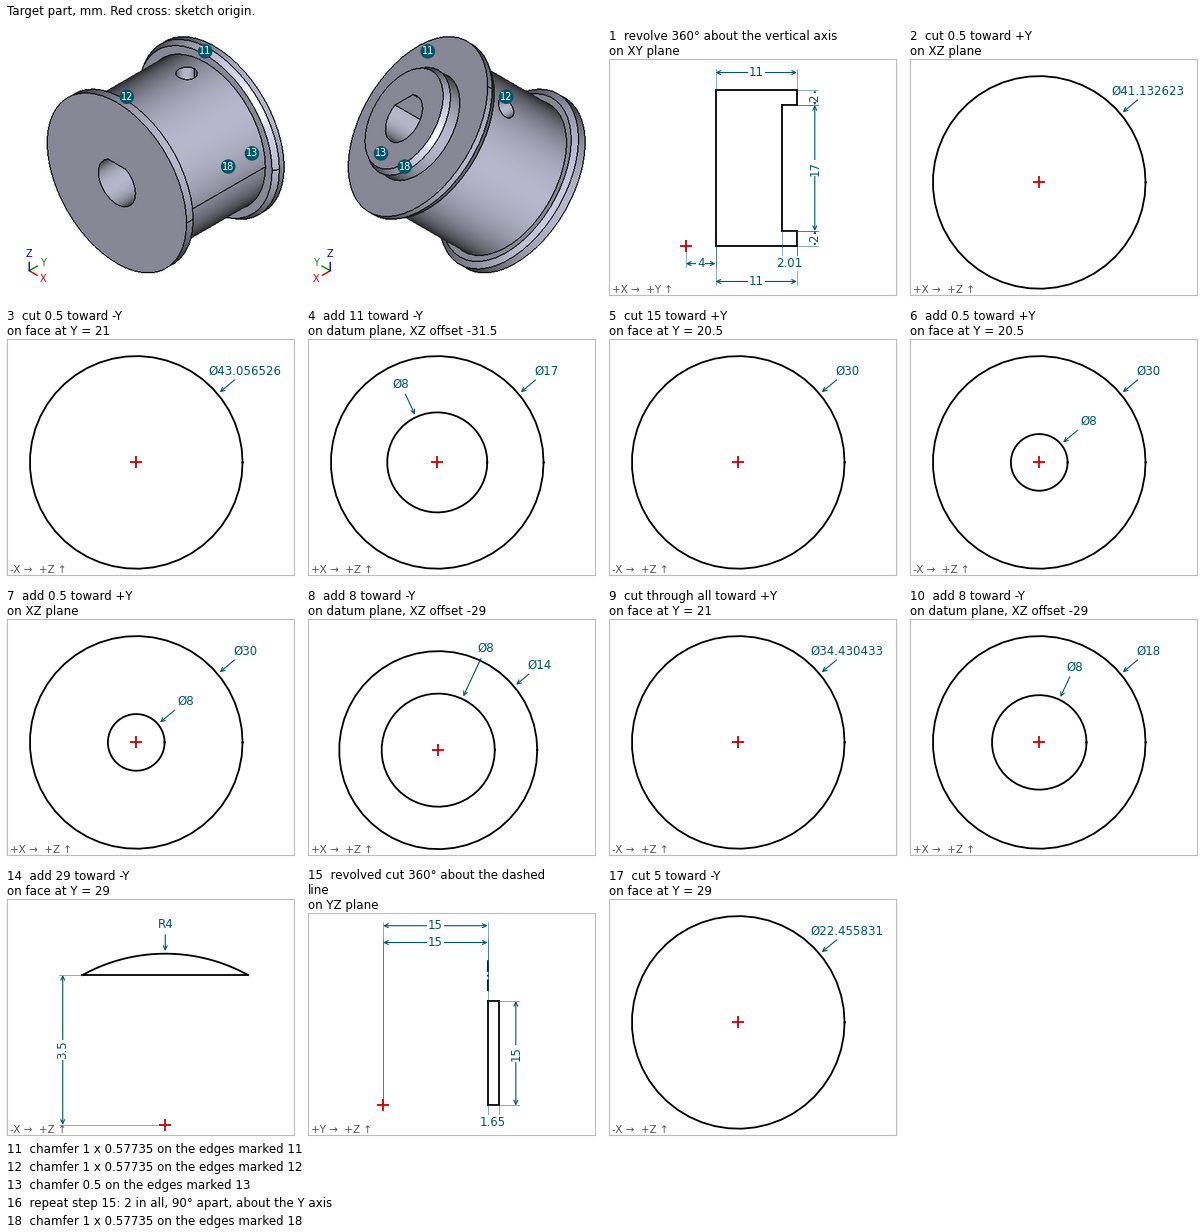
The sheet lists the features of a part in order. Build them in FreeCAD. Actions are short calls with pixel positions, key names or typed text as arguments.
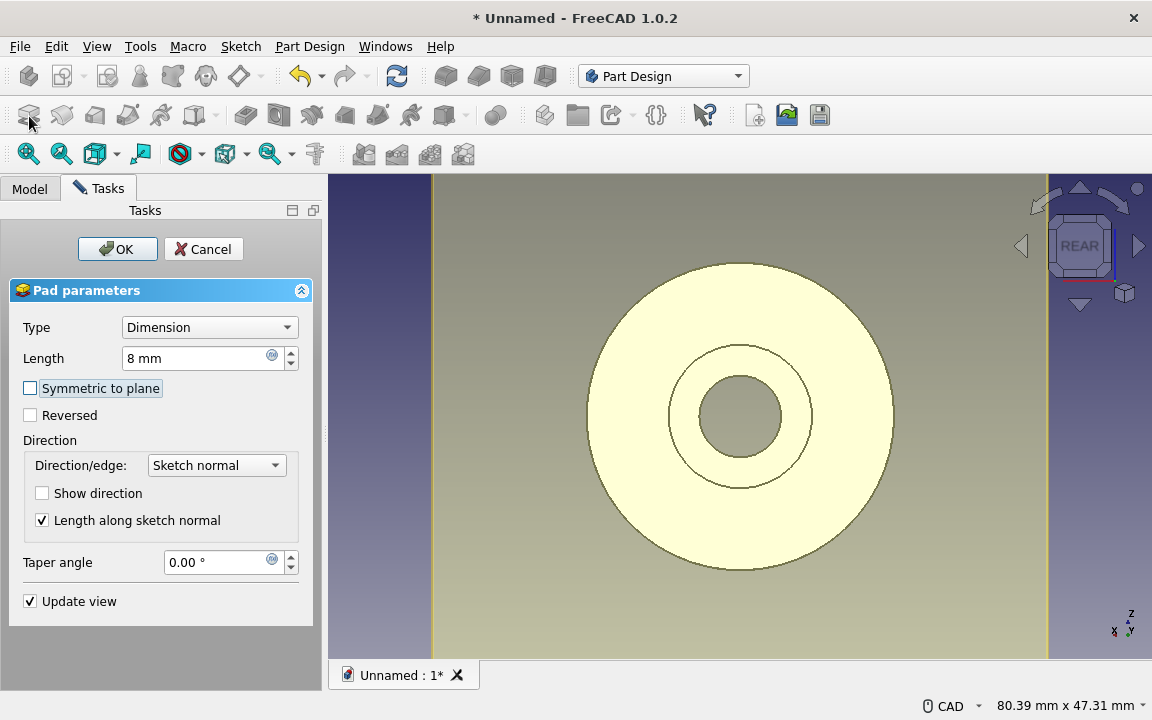
click(118, 249)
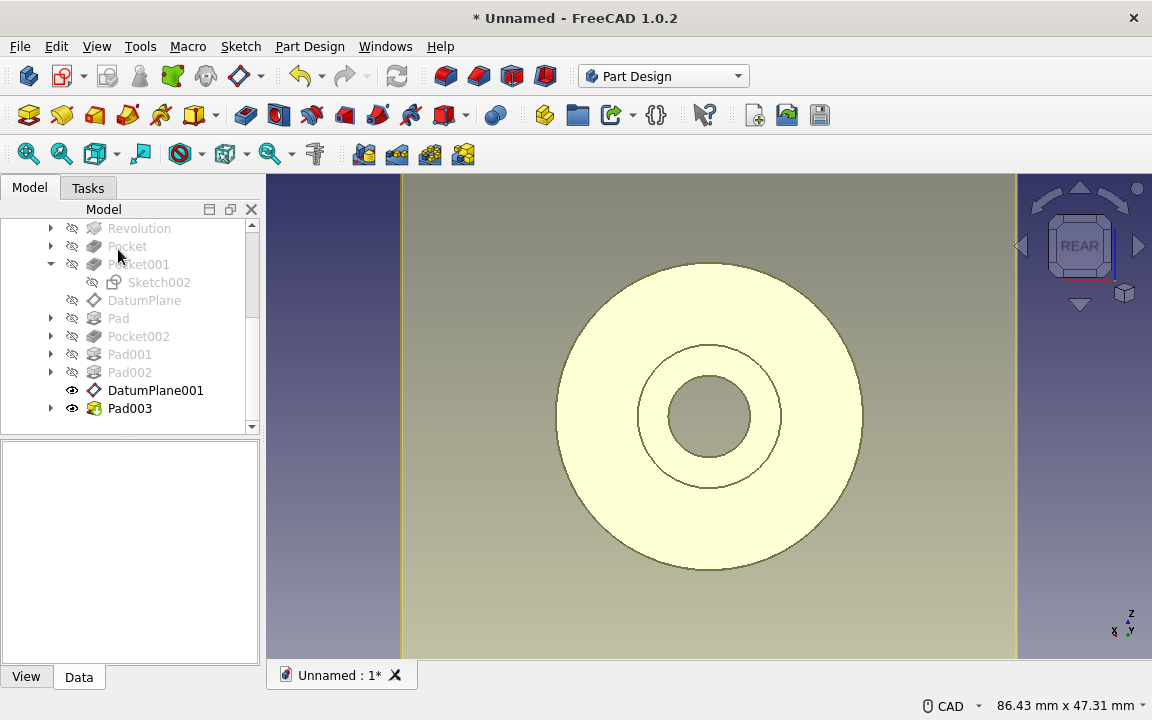
click(117, 390)
key(space)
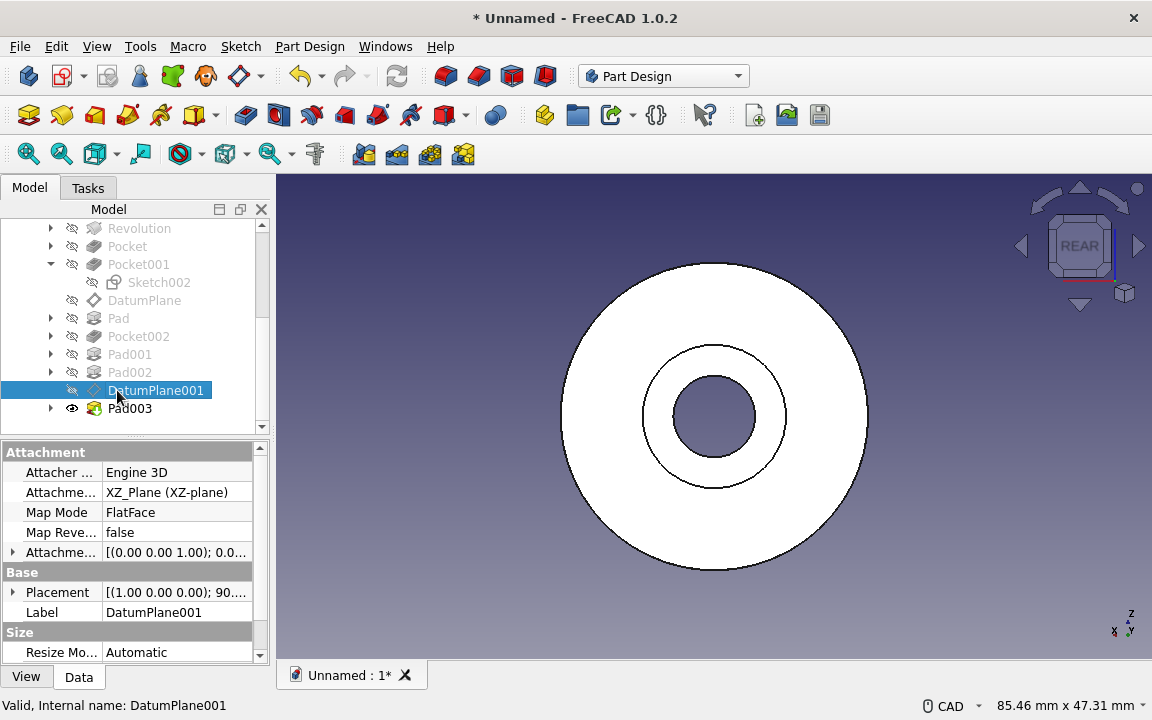
click(802, 503)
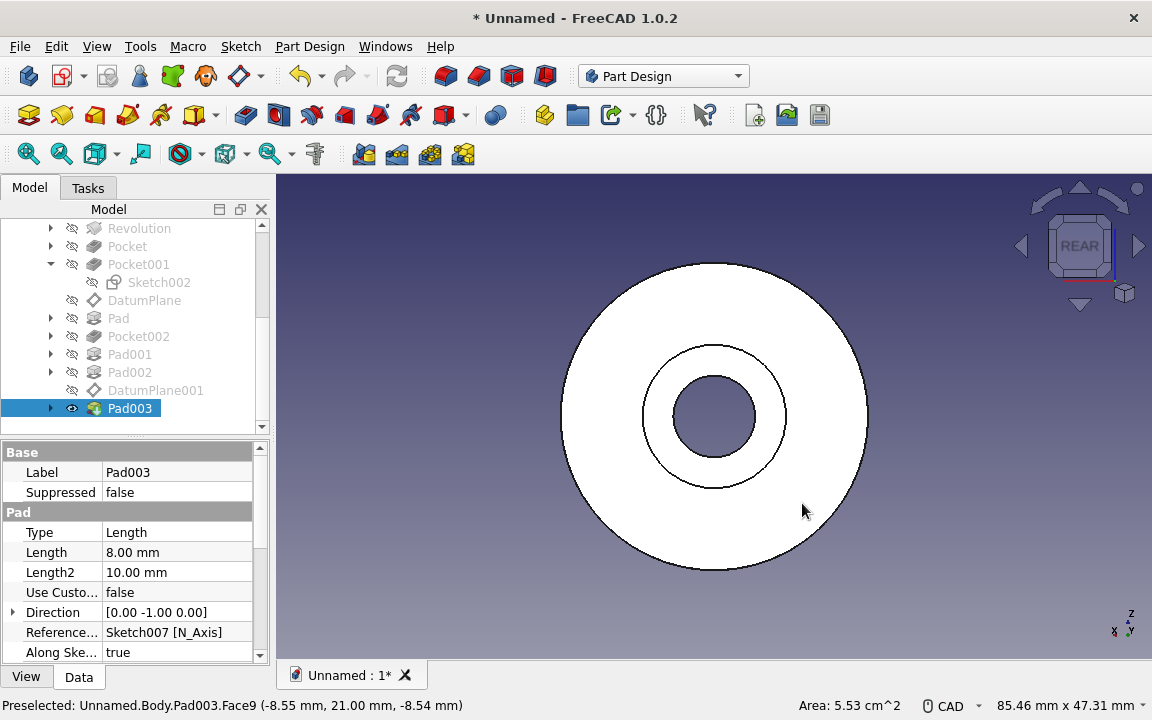
click(62, 76)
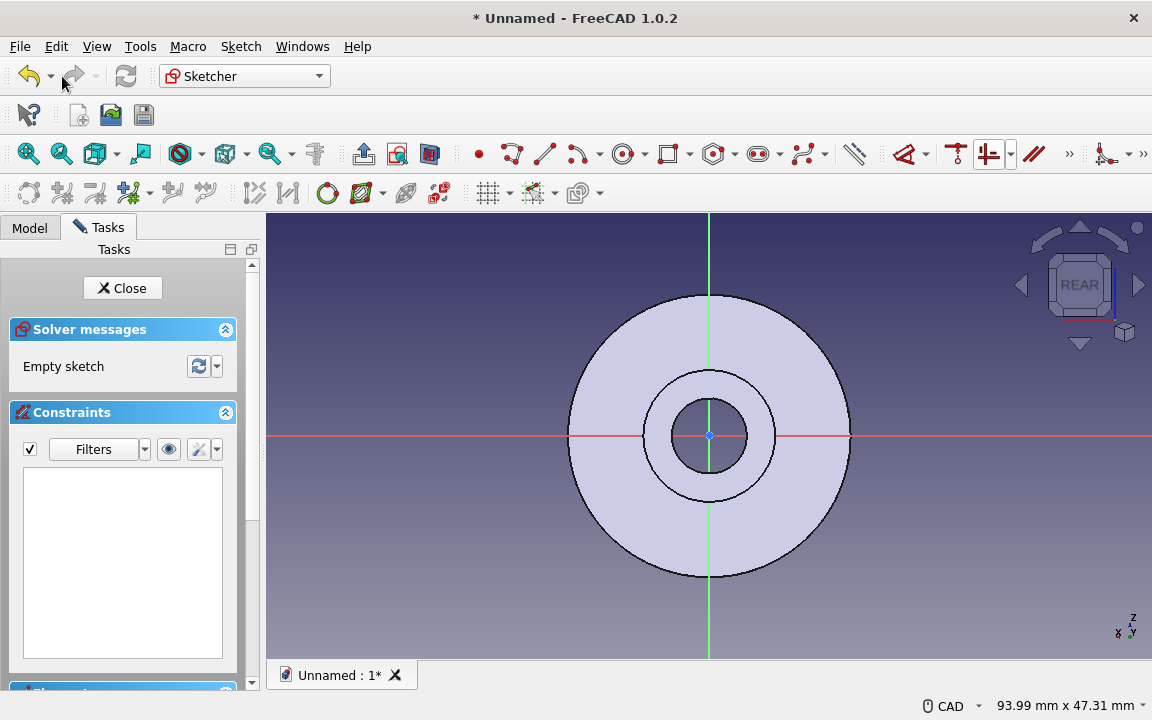
click(622, 154)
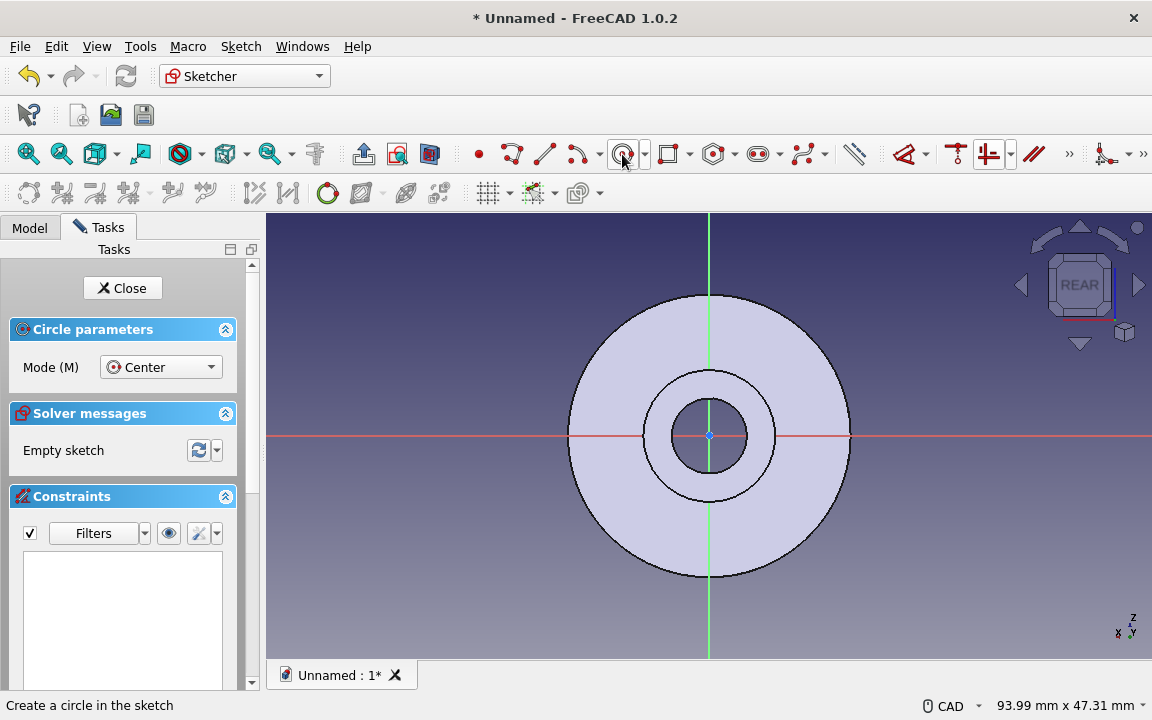
click(709, 436)
move(824, 321)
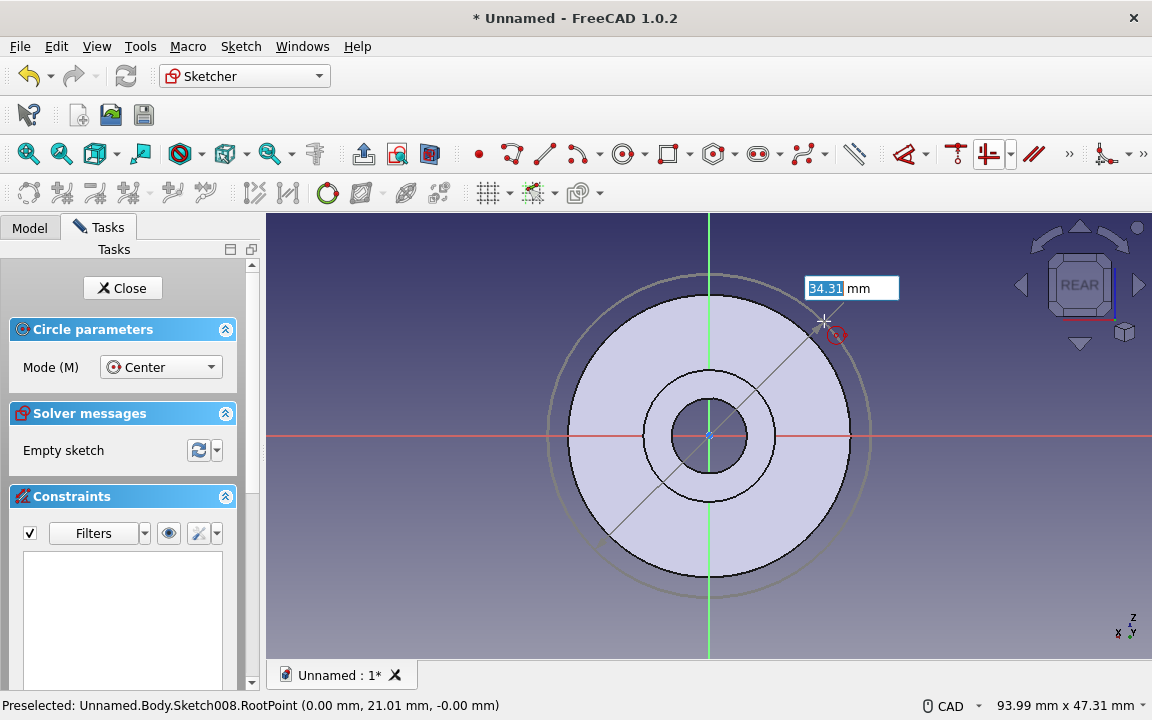
text(34.430433)
key(Return)
key(Escape)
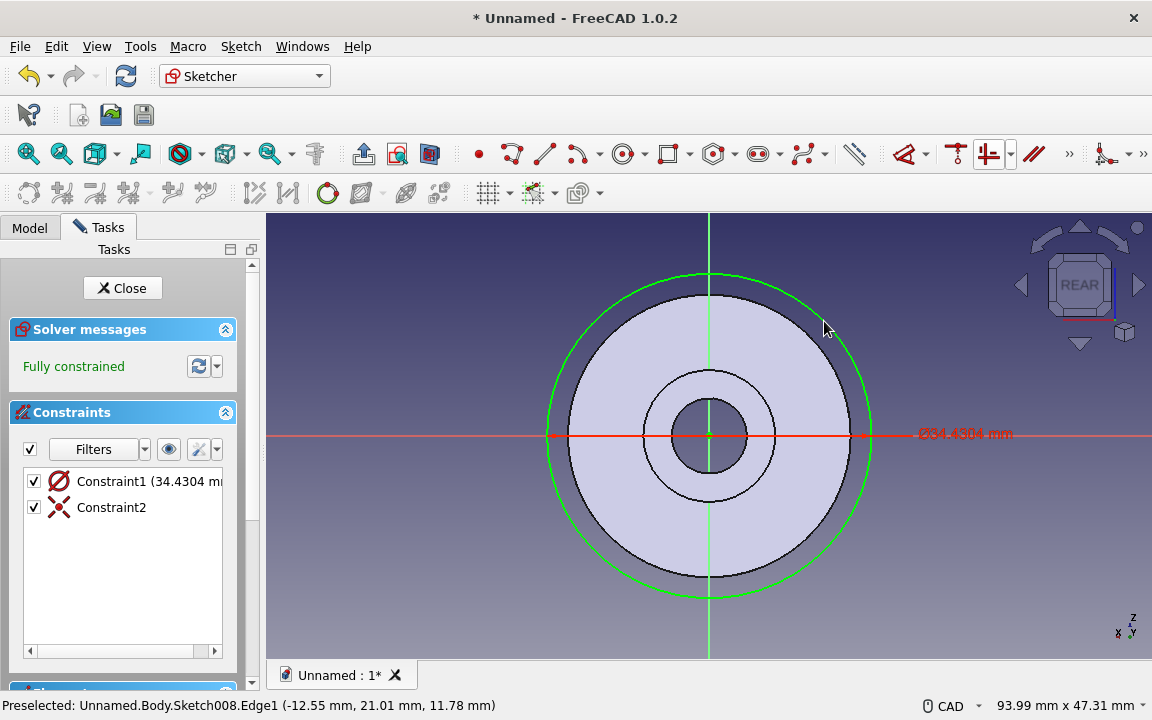
click(123, 288)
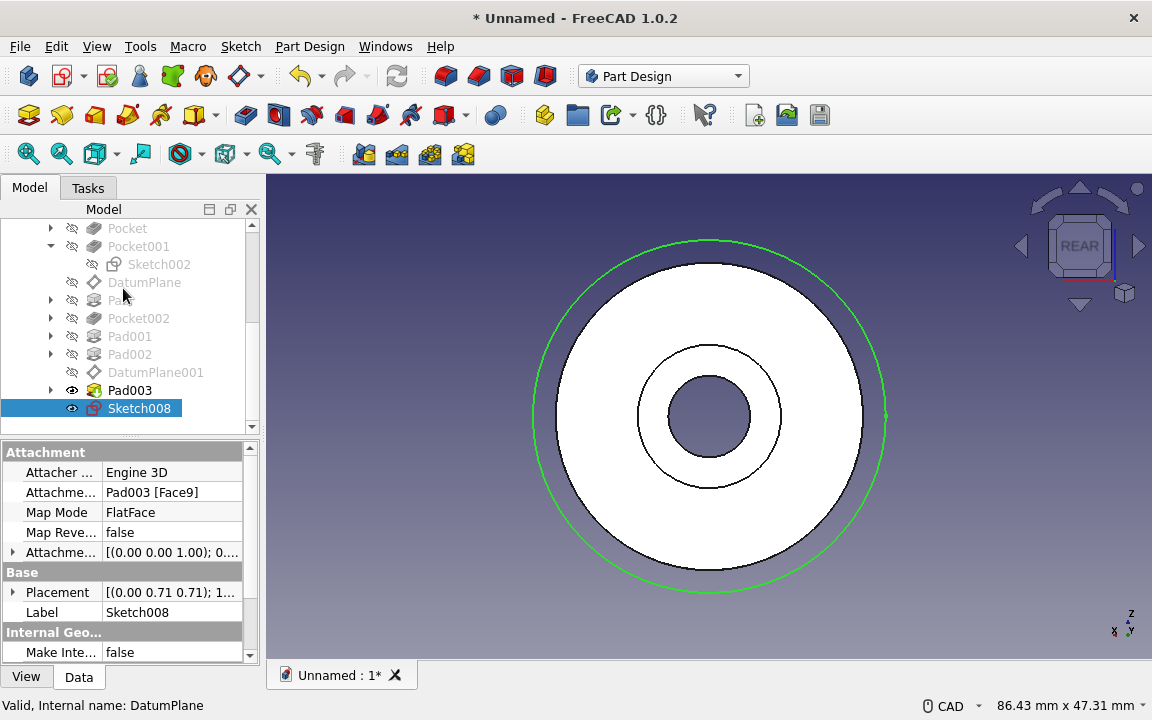
click(246, 116)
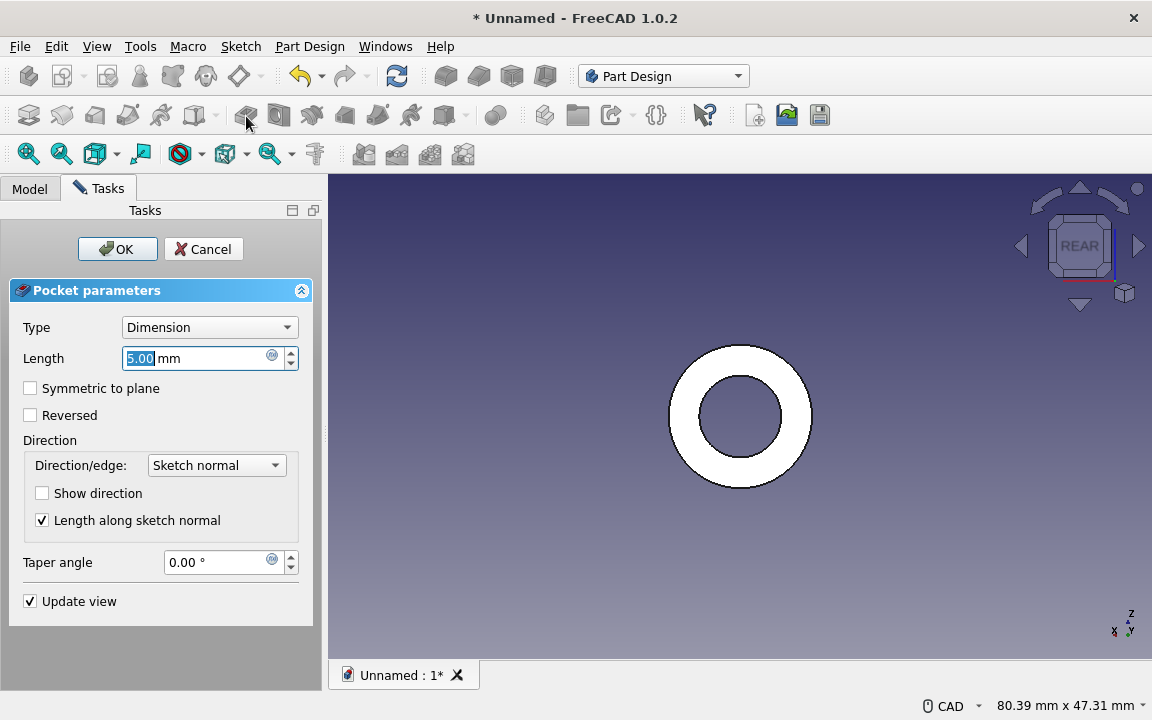
click(210, 328)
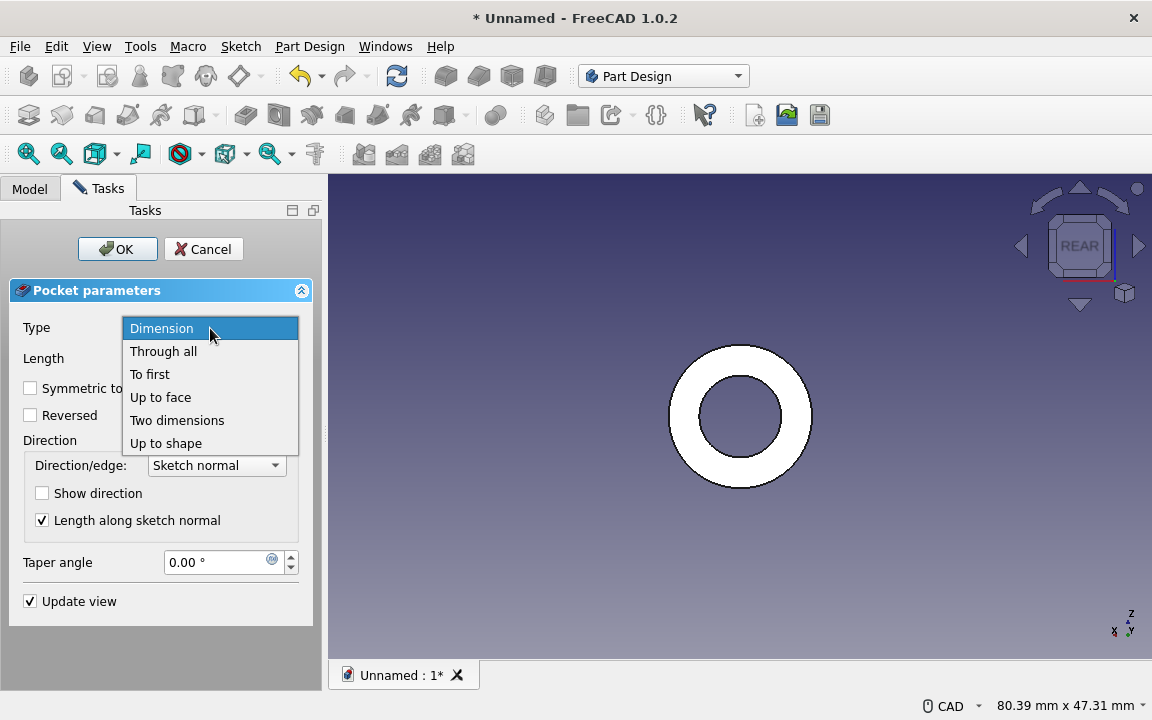
click(208, 352)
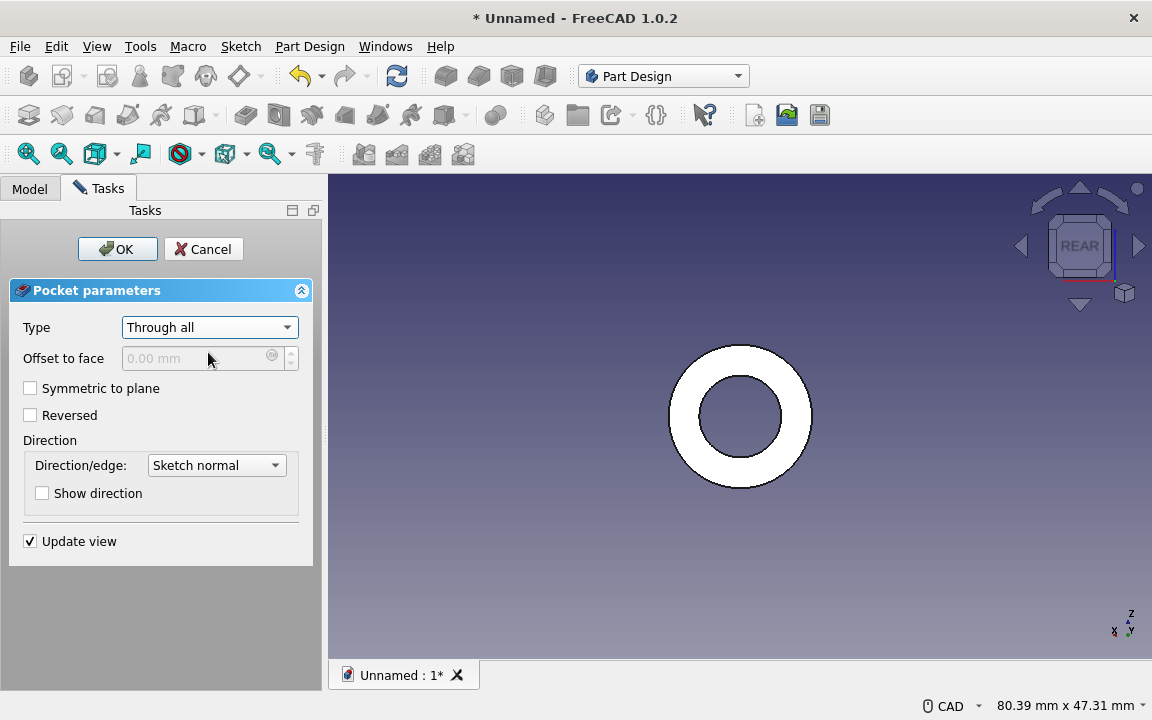
click(31, 415)